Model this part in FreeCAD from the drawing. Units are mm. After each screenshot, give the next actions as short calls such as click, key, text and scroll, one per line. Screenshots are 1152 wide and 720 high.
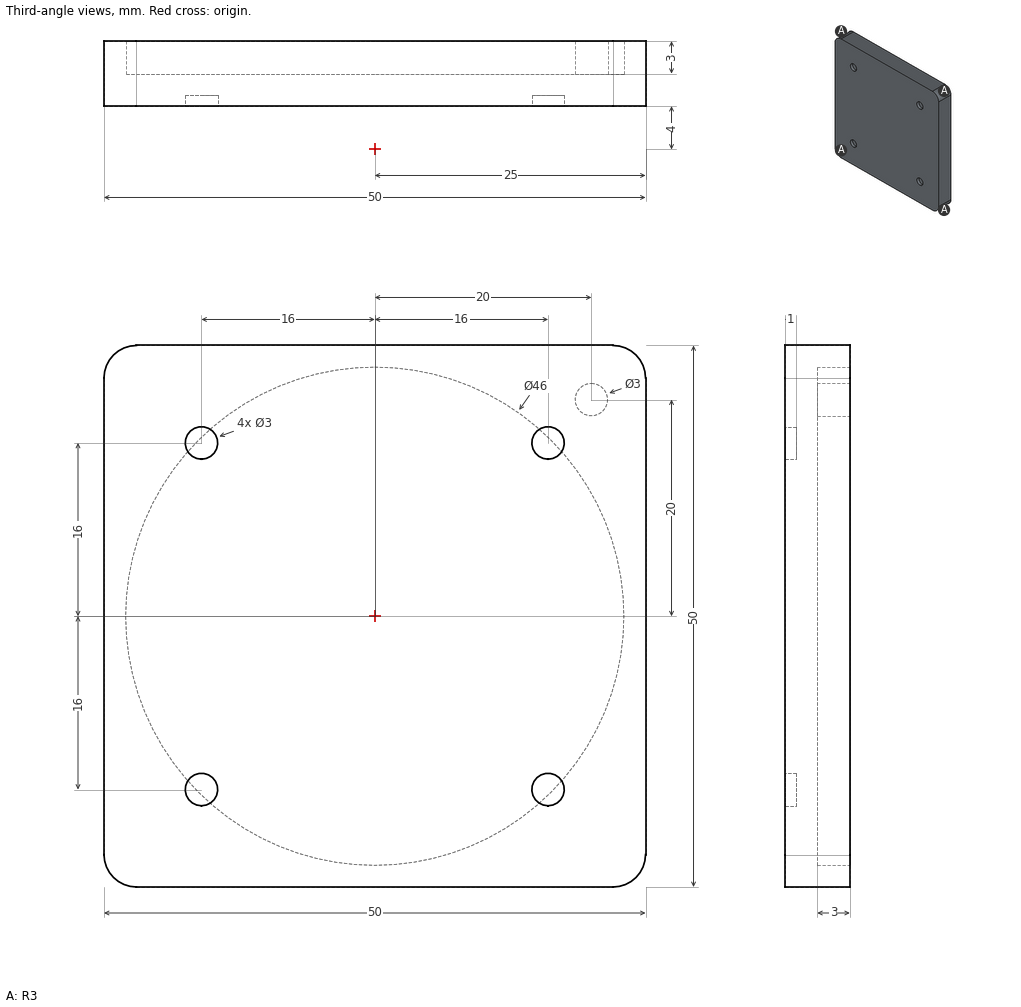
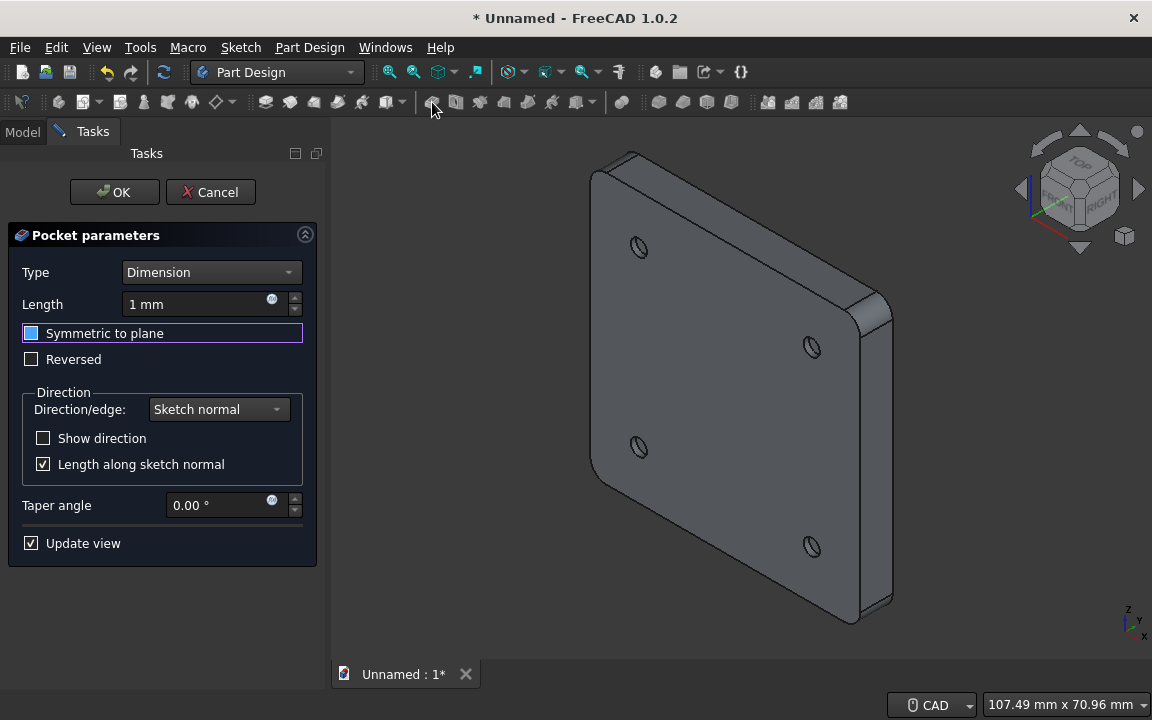
click(115, 192)